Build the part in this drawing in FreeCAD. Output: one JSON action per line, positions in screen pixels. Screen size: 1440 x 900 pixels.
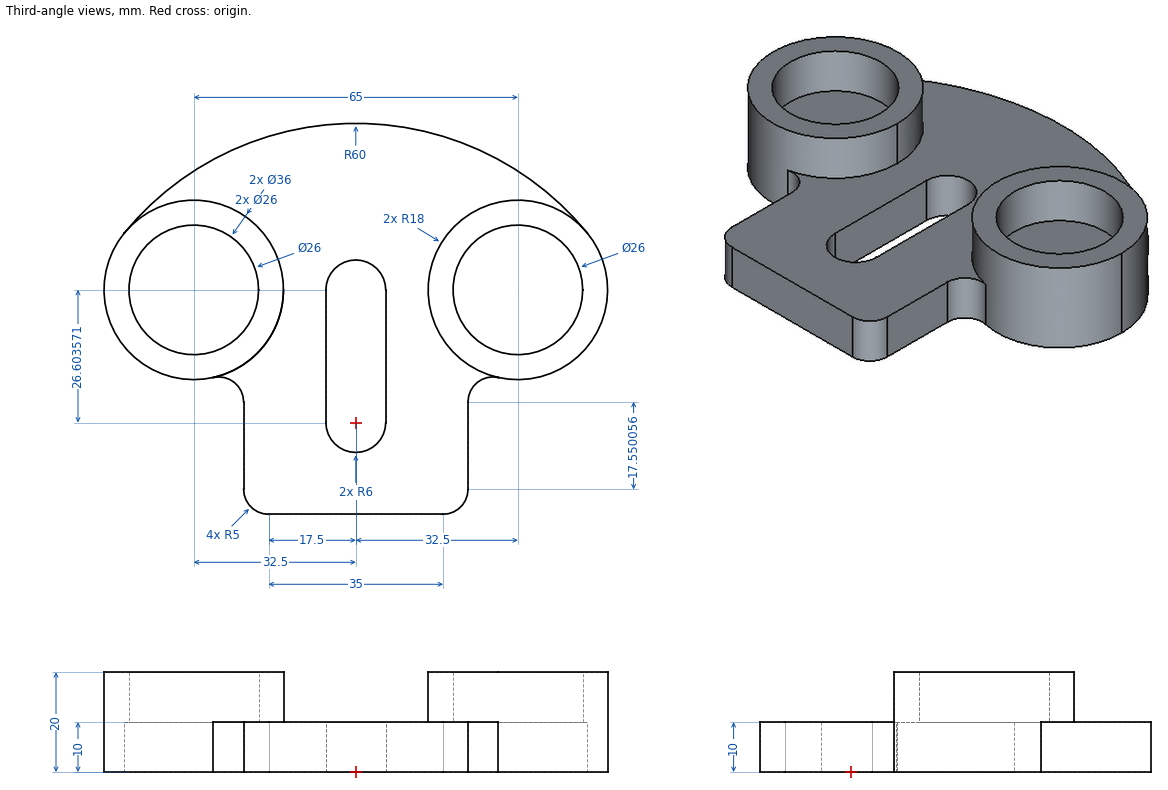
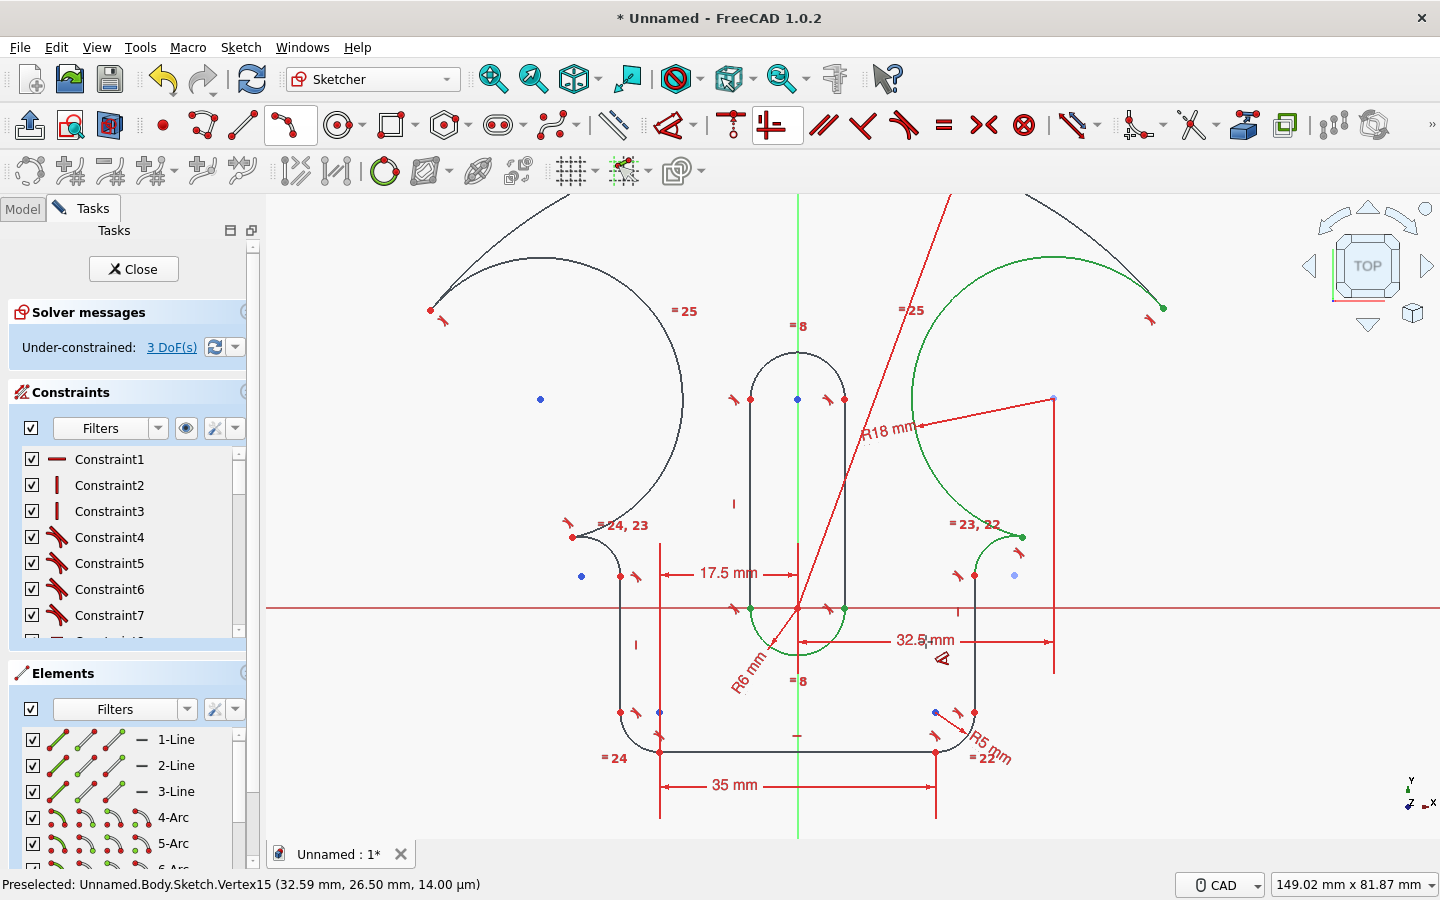
{"action": "left_click", "coordinate": [541, 399]}
{"action": "left_click", "coordinate": [669, 642]}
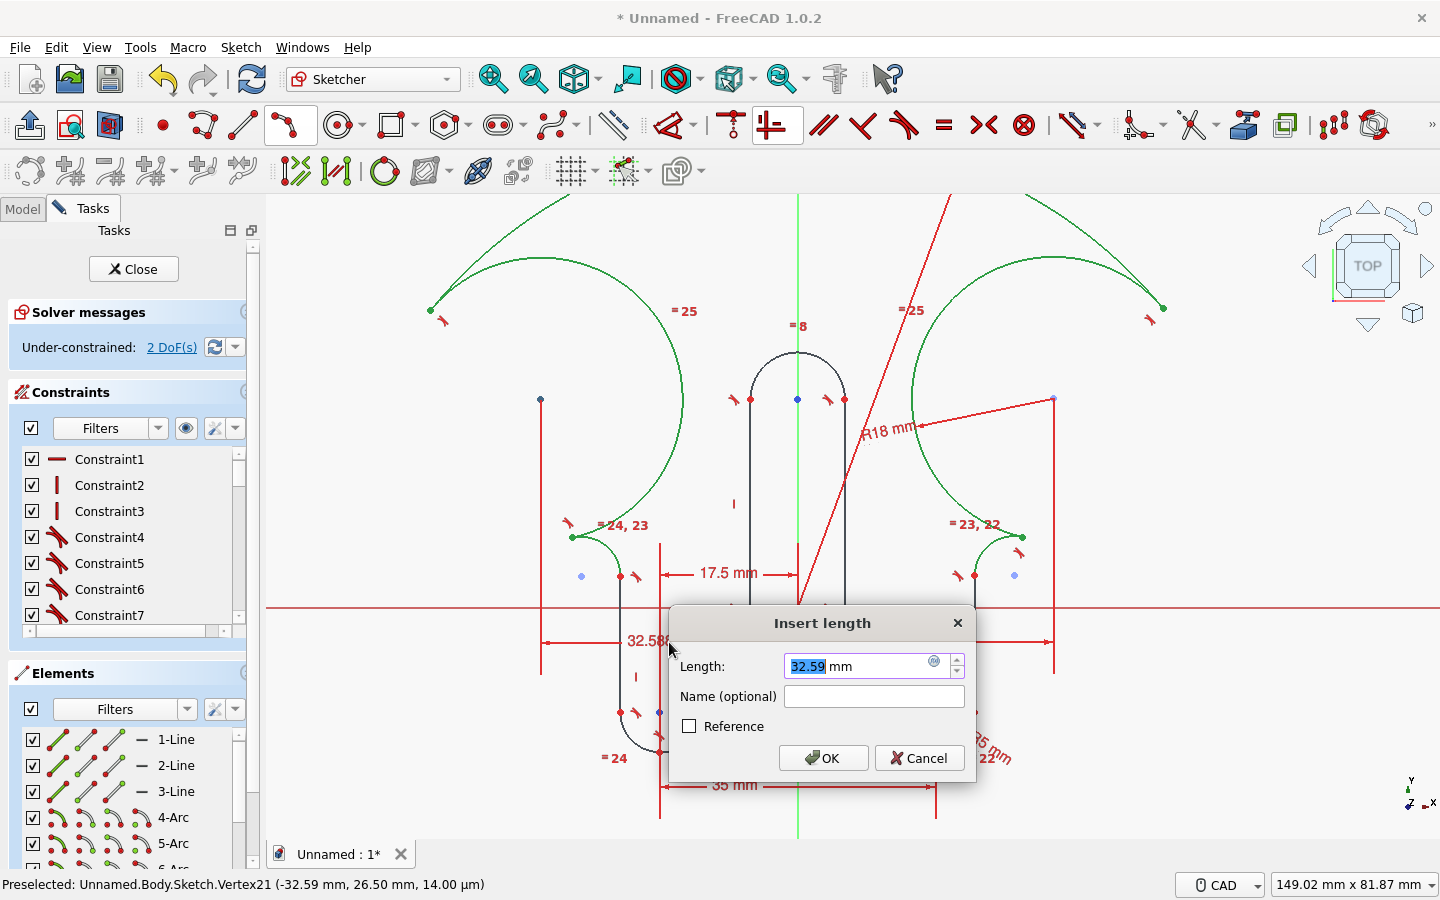
{"action": "type", "text": "32.5"}
{"action": "key", "text": "Return"}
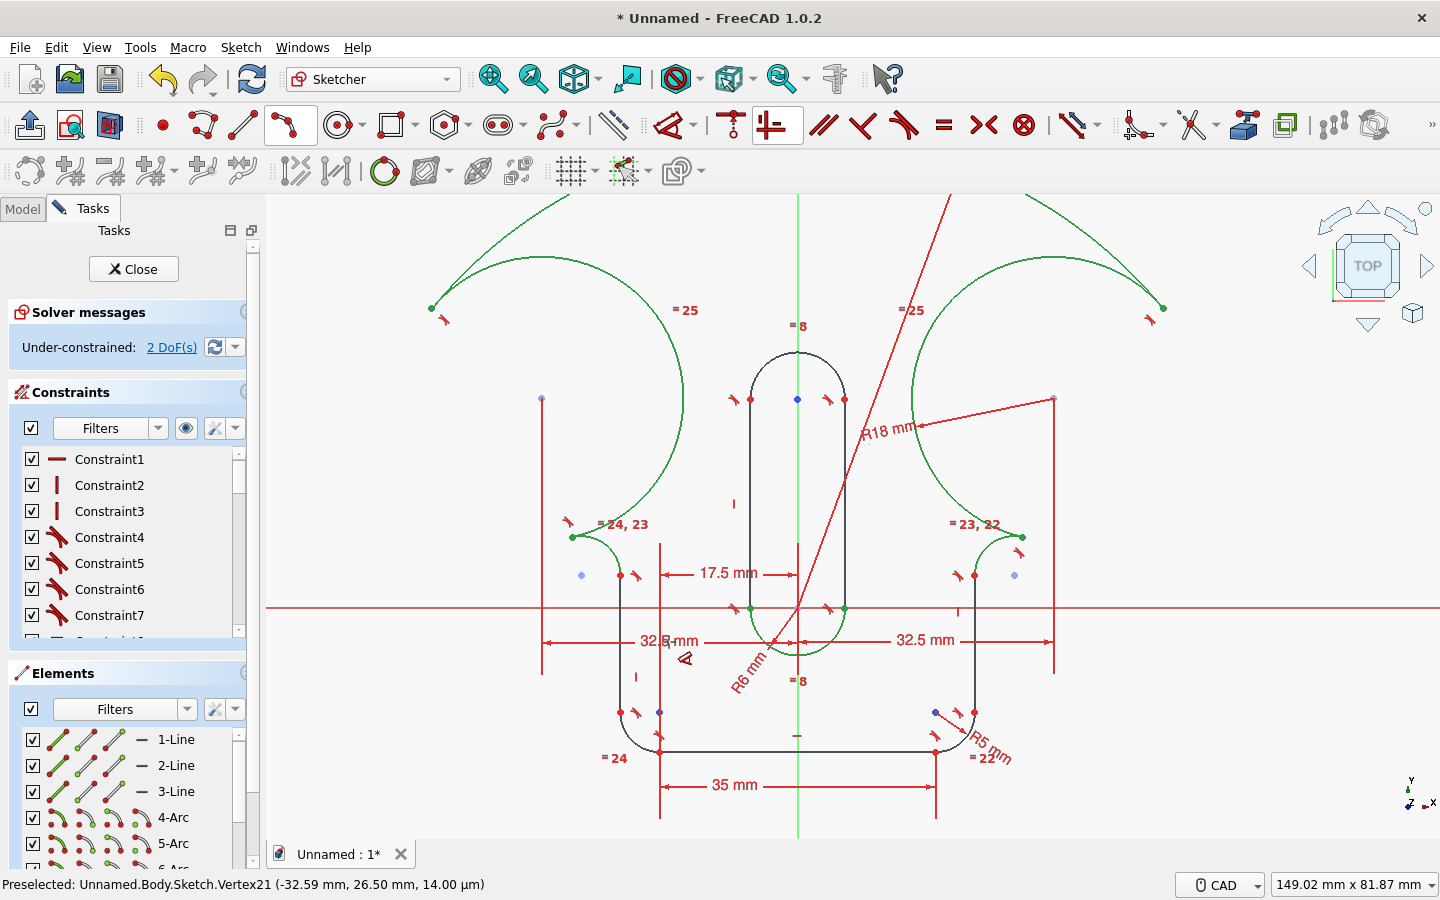
{"action": "left_click", "coordinate": [975, 672]}
{"action": "left_click", "coordinate": [1009, 644]}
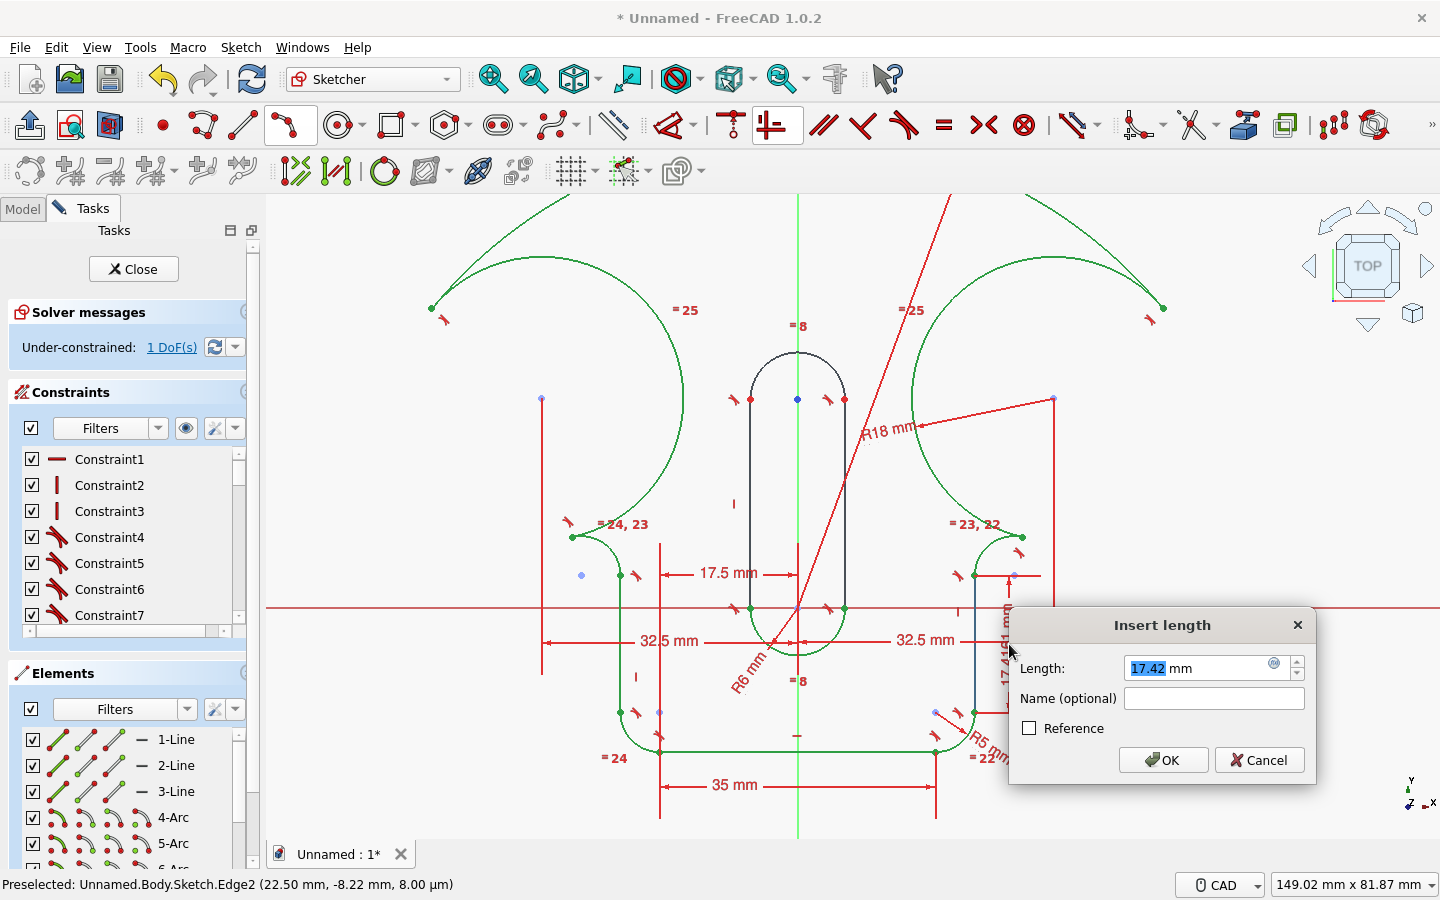
{"action": "type", "text": "17.550056"}
{"action": "key", "text": "Return"}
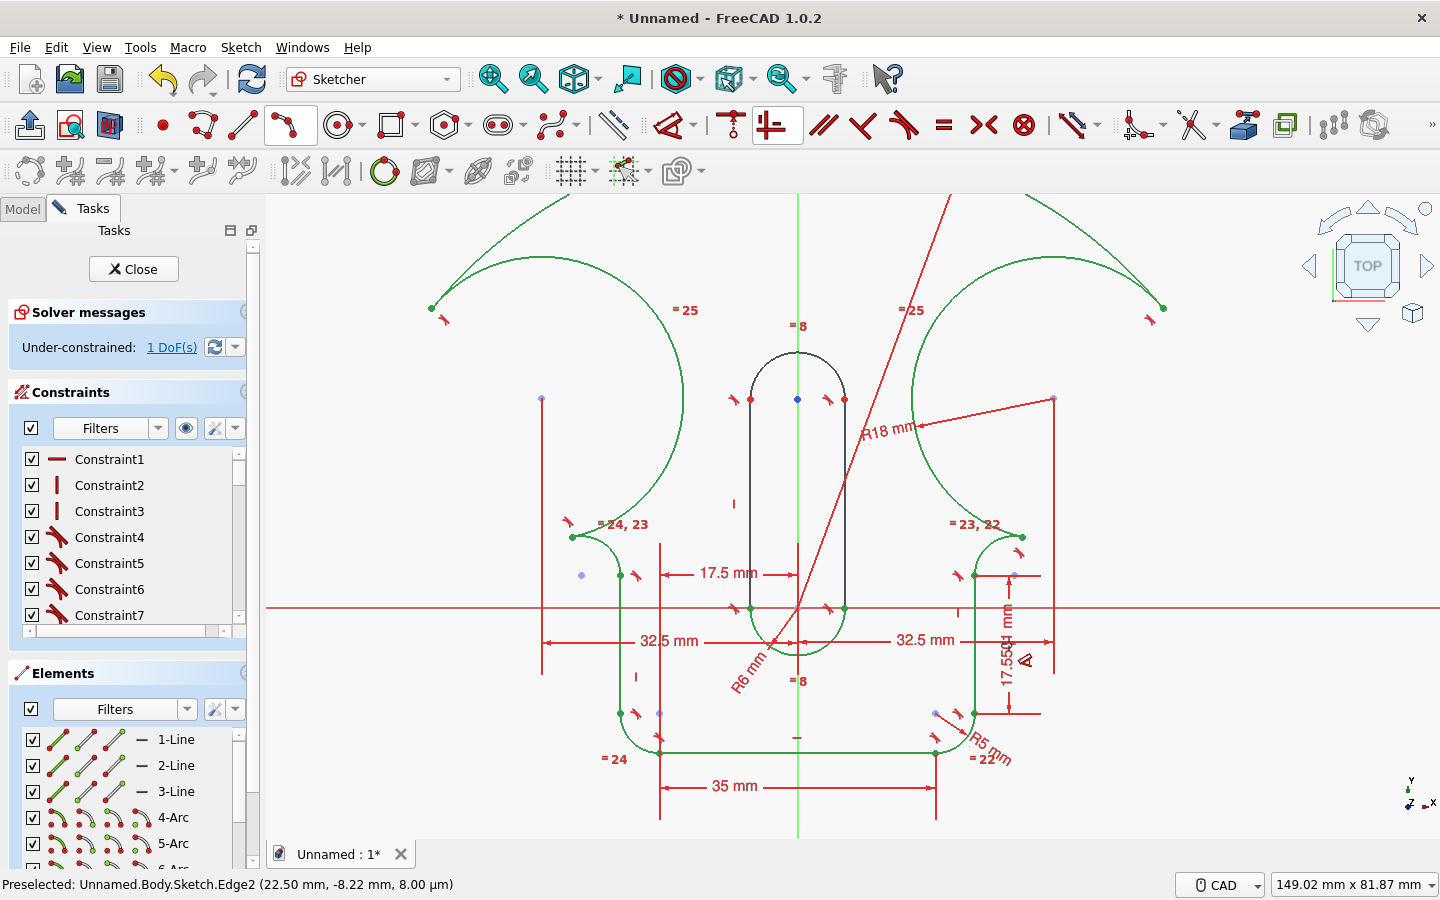
{"action": "left_click", "coordinate": [750, 546]}
{"action": "left_click", "coordinate": [716, 504]}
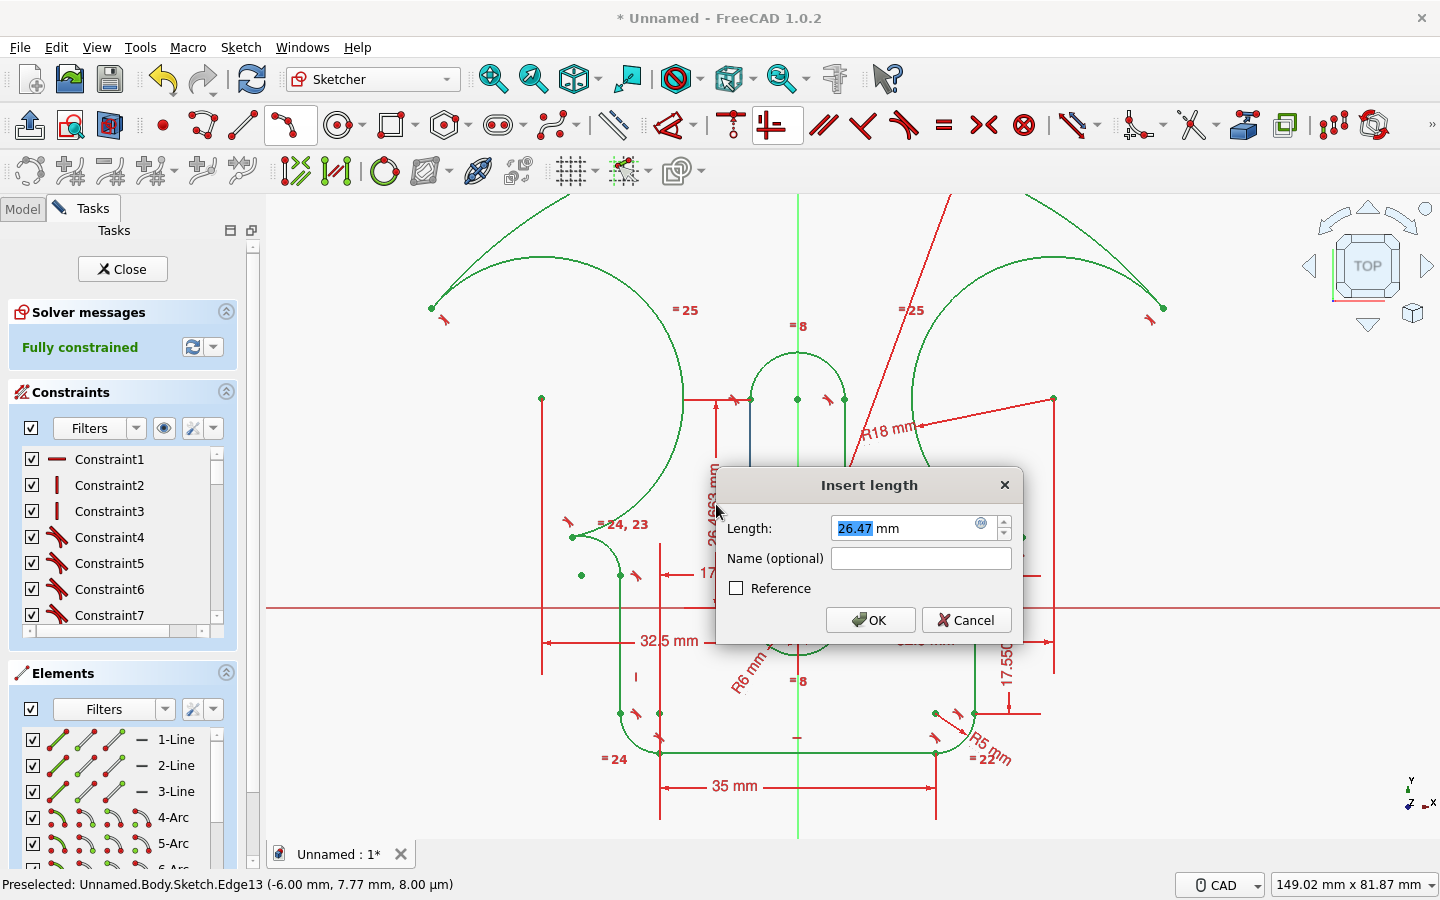
{"action": "type", "text": "26.603571"}
{"action": "key", "text": "Return"}
{"action": "key", "text": "Escape"}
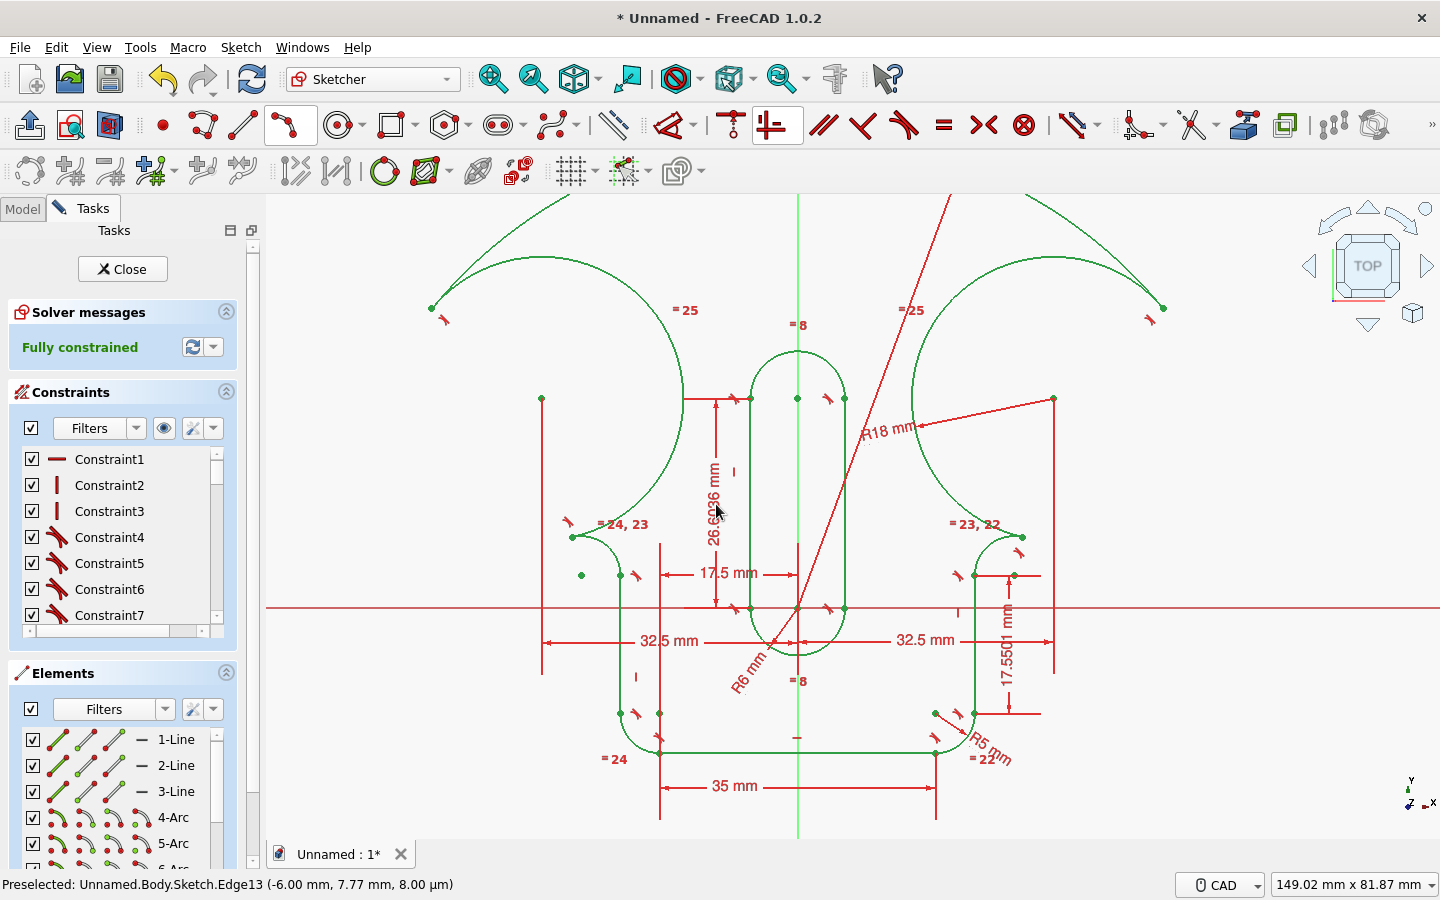
{"action": "left_click", "coordinate": [123, 269]}